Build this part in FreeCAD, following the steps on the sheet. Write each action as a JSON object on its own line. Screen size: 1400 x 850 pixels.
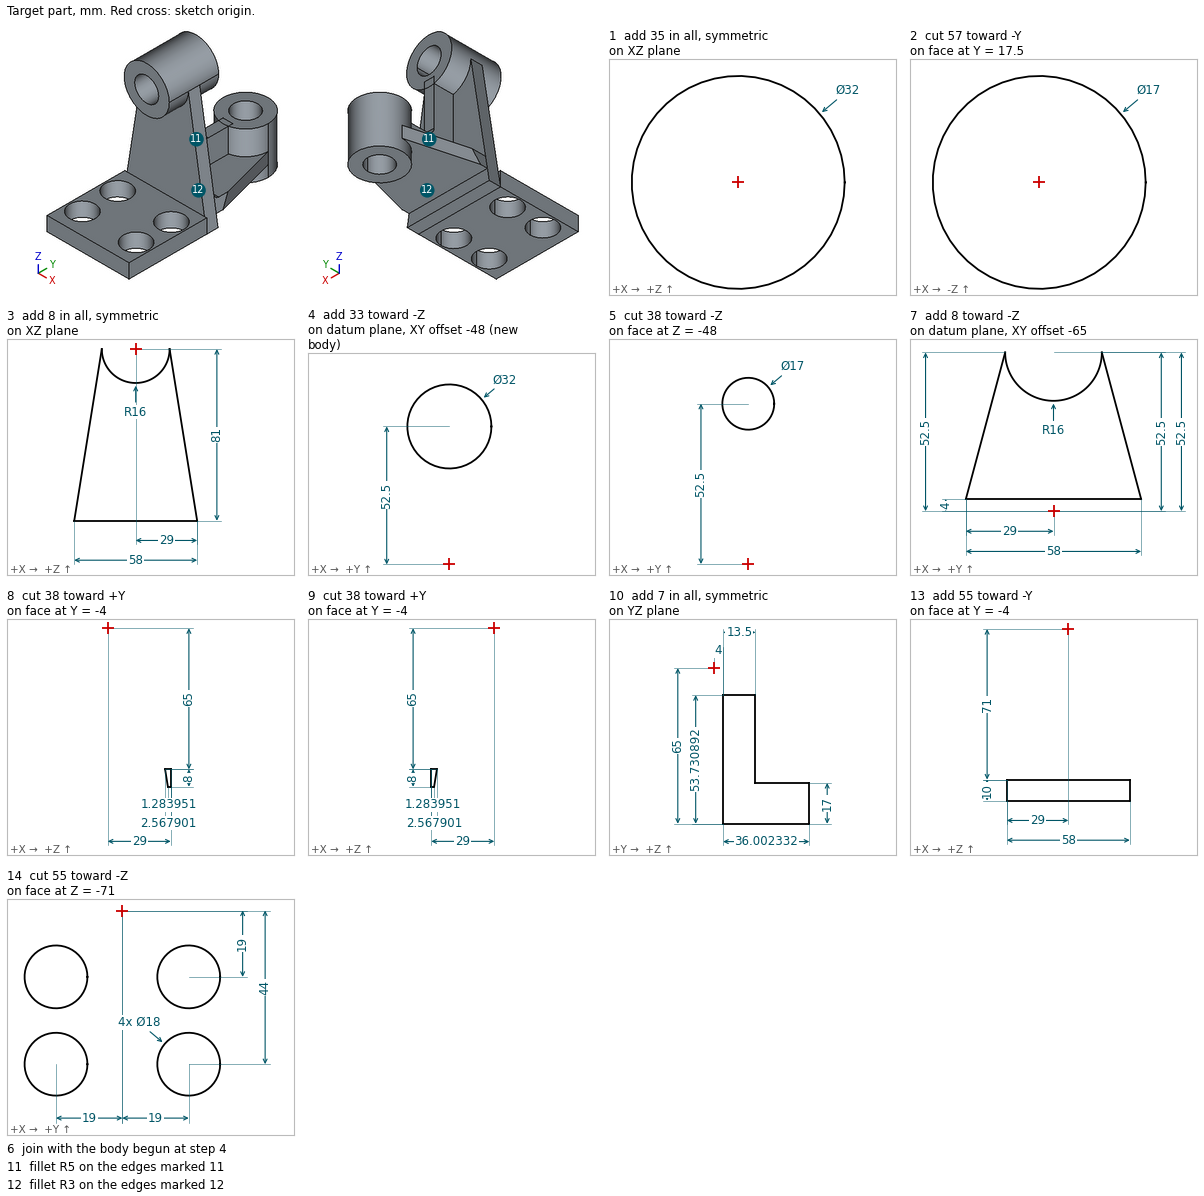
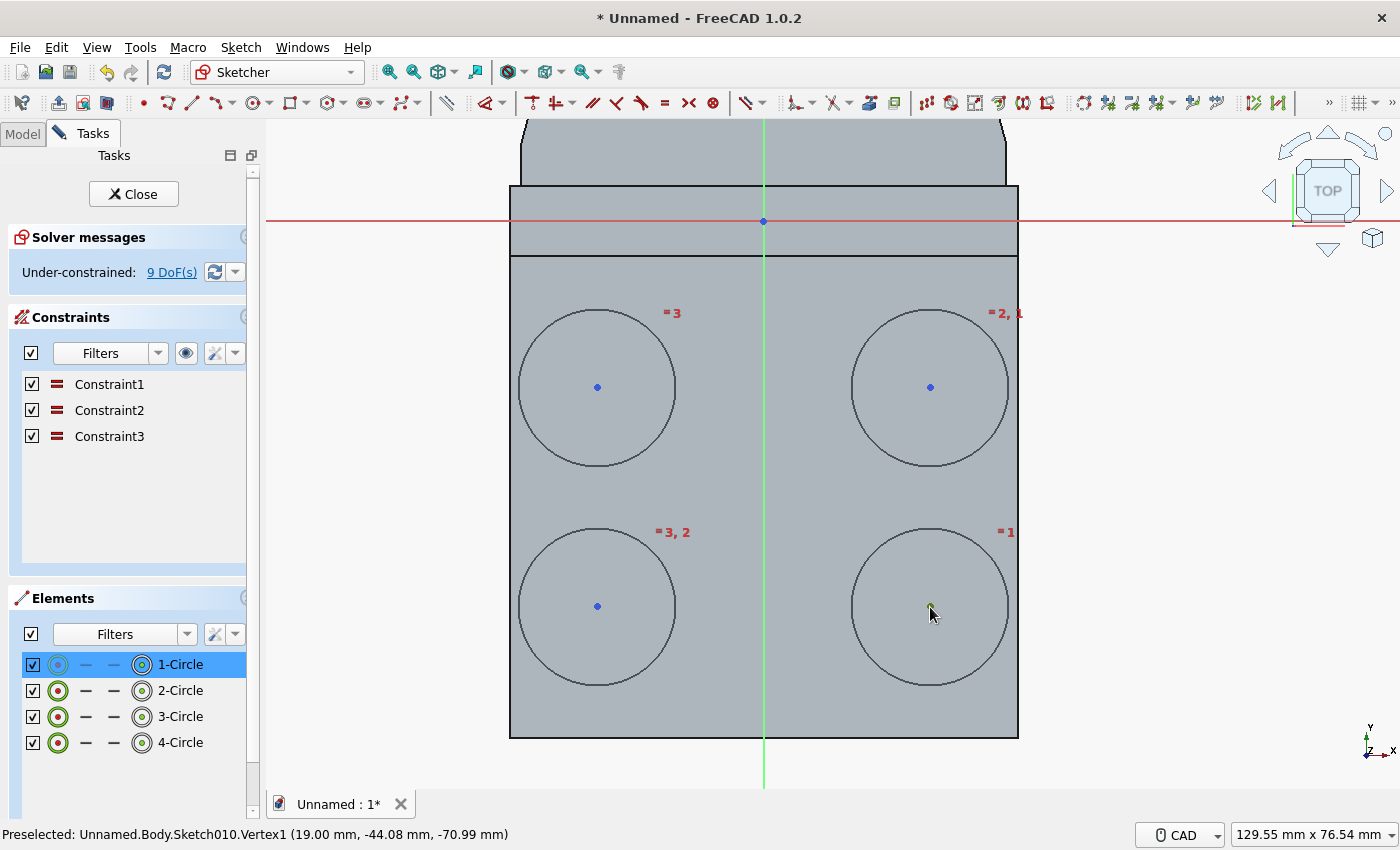
{"action": "left_click", "coordinate": [930, 388]}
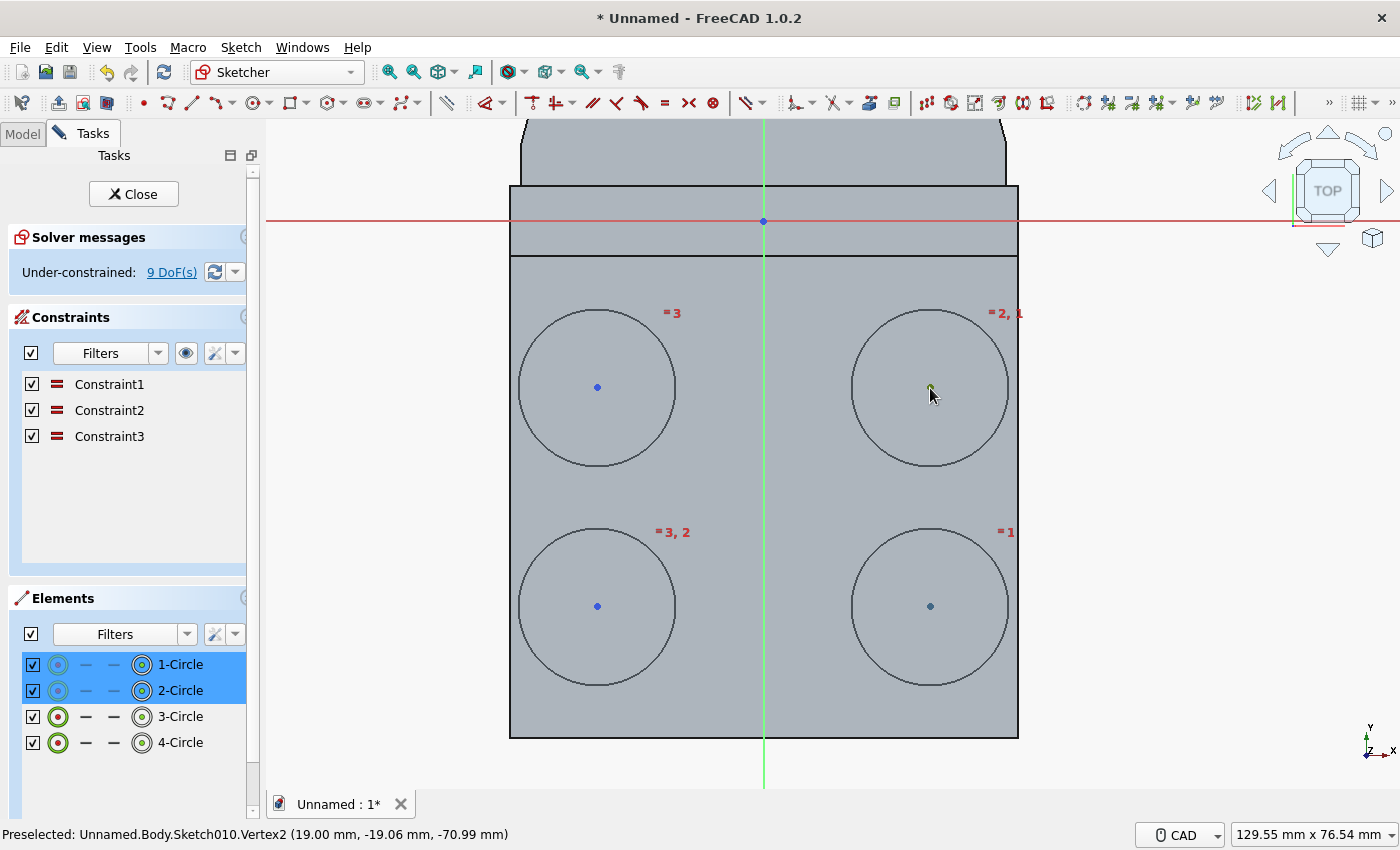
{"action": "left_click", "coordinate": [574, 104]}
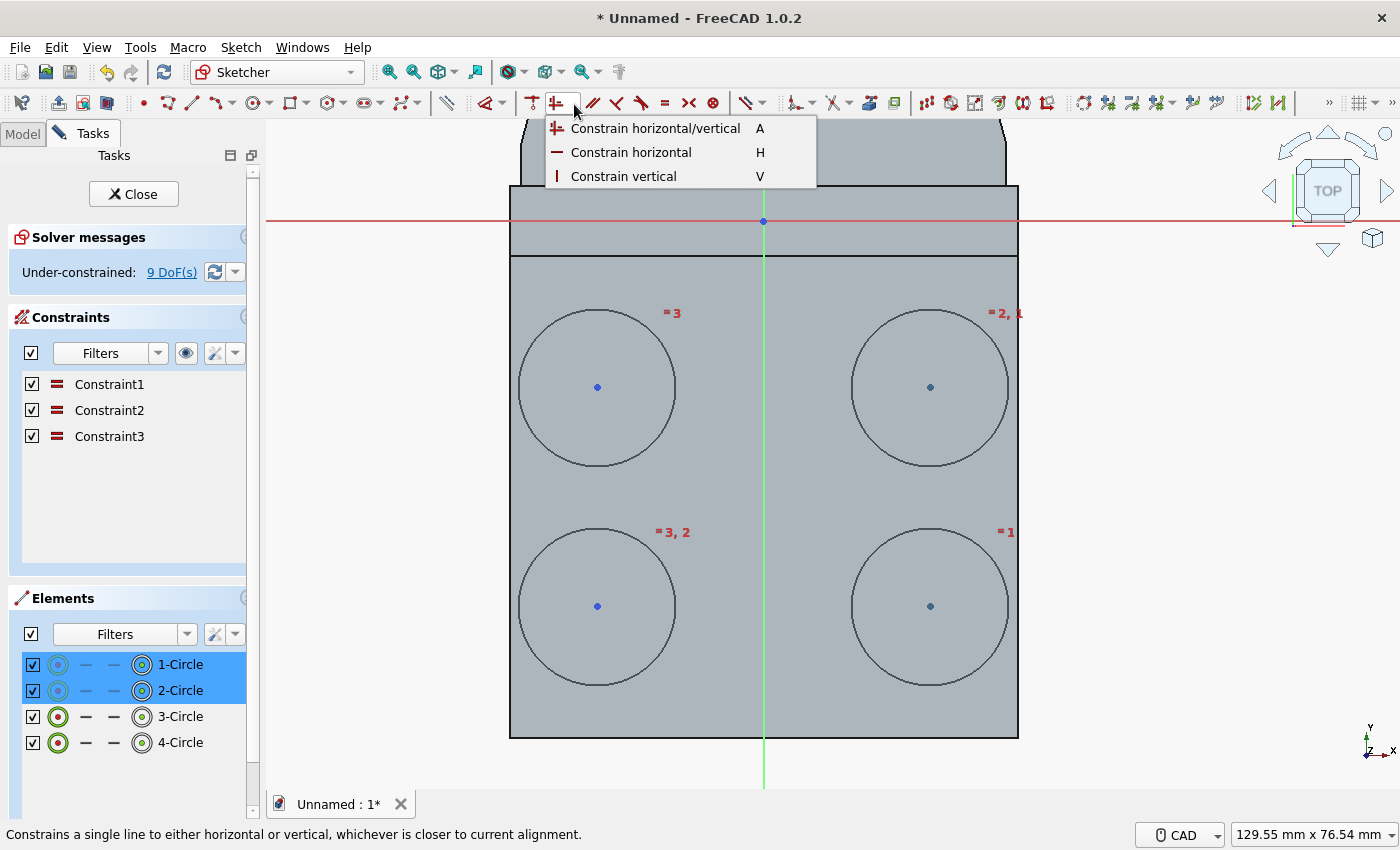
{"action": "left_click", "coordinate": [681, 176]}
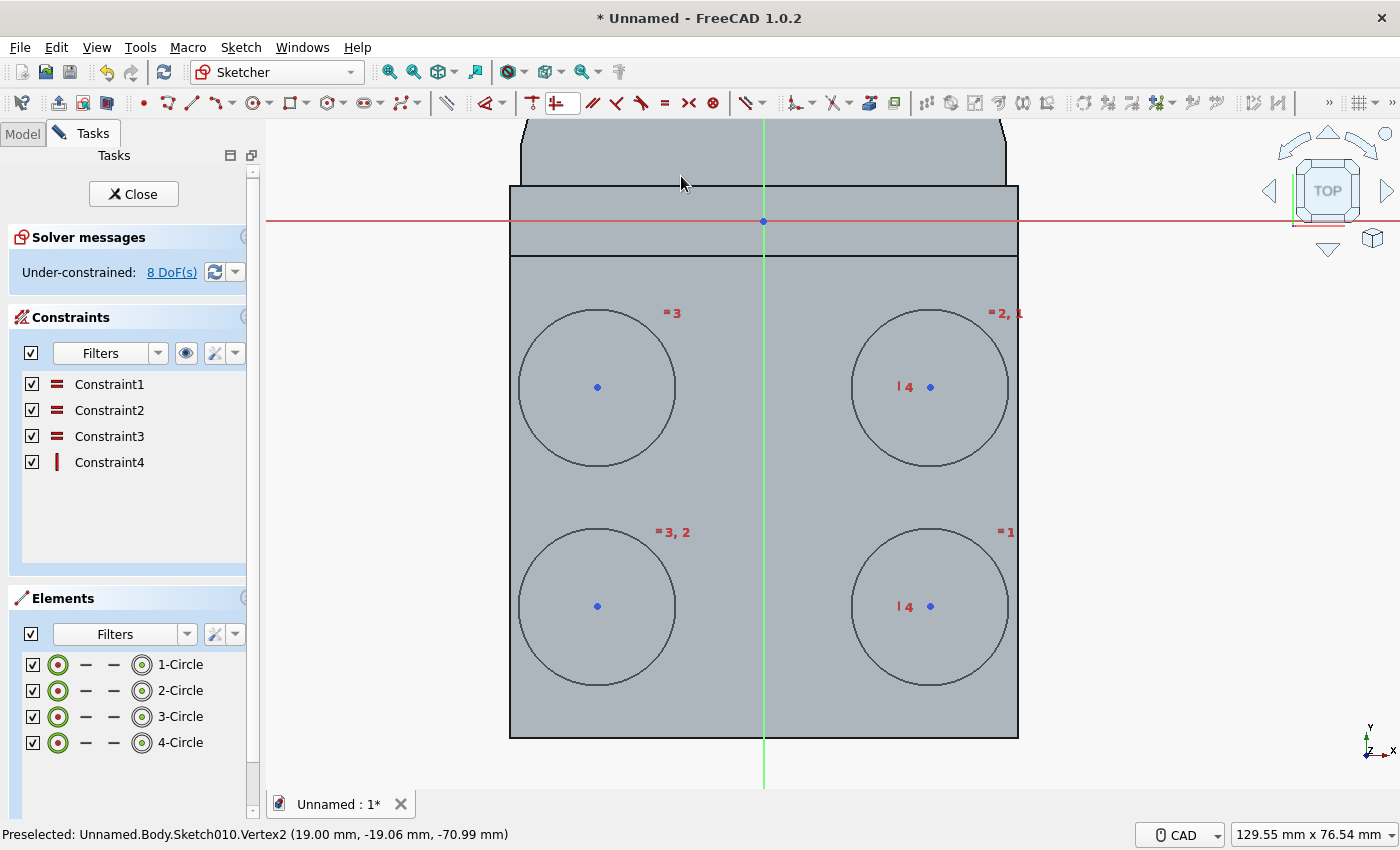
{"action": "left_click", "coordinate": [930, 607]}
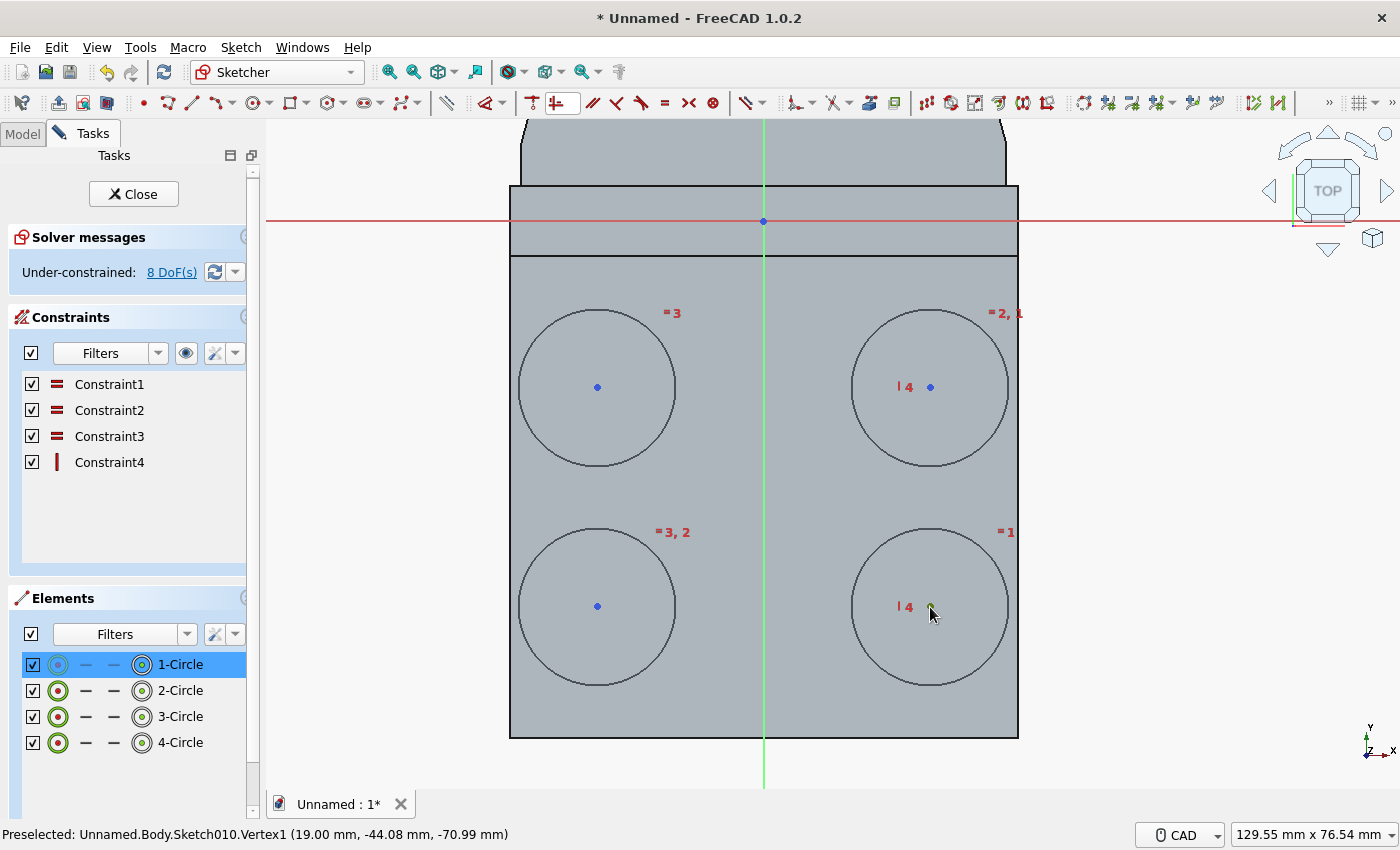
{"action": "left_click", "coordinate": [597, 607]}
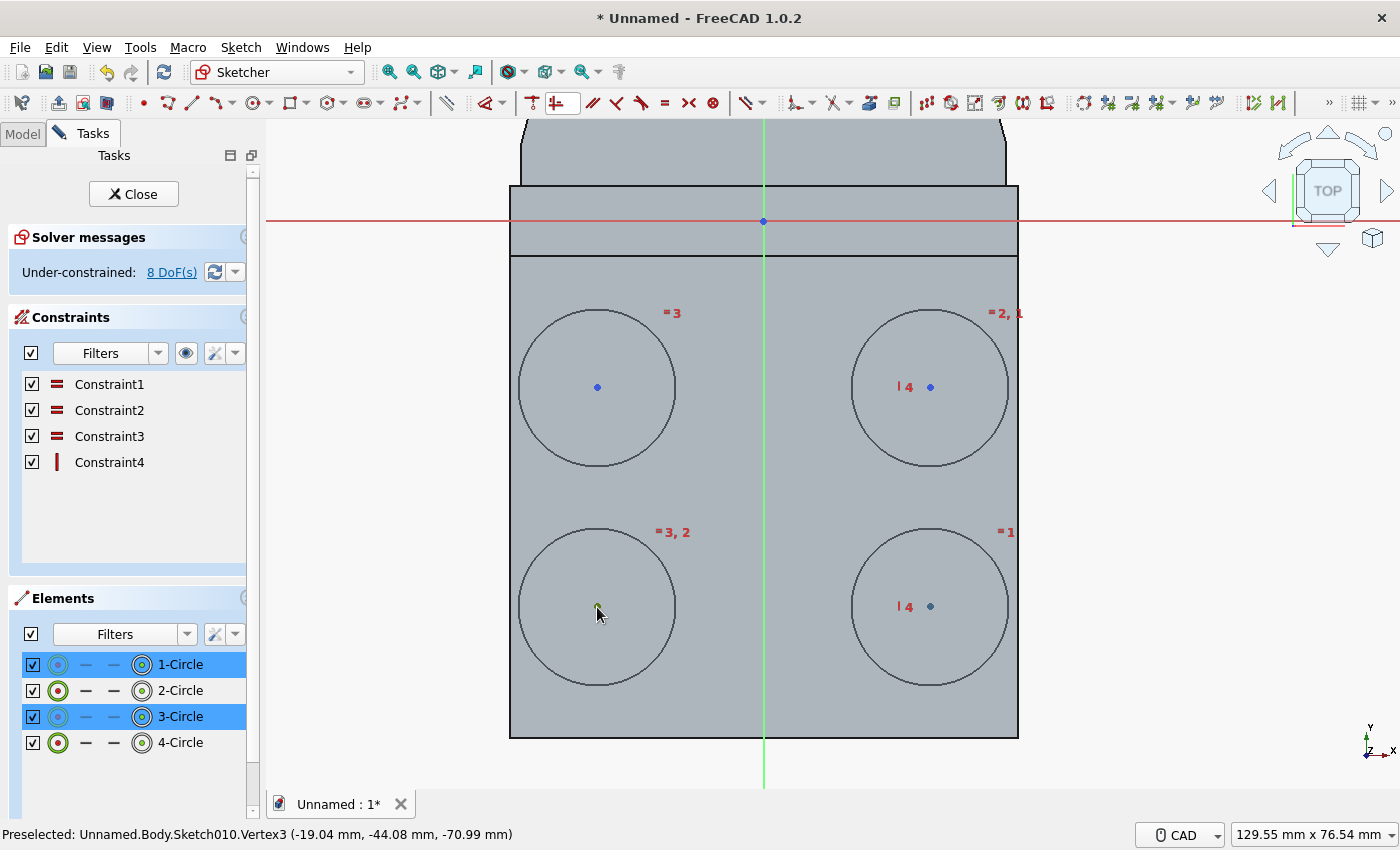
{"action": "key", "text": "h"}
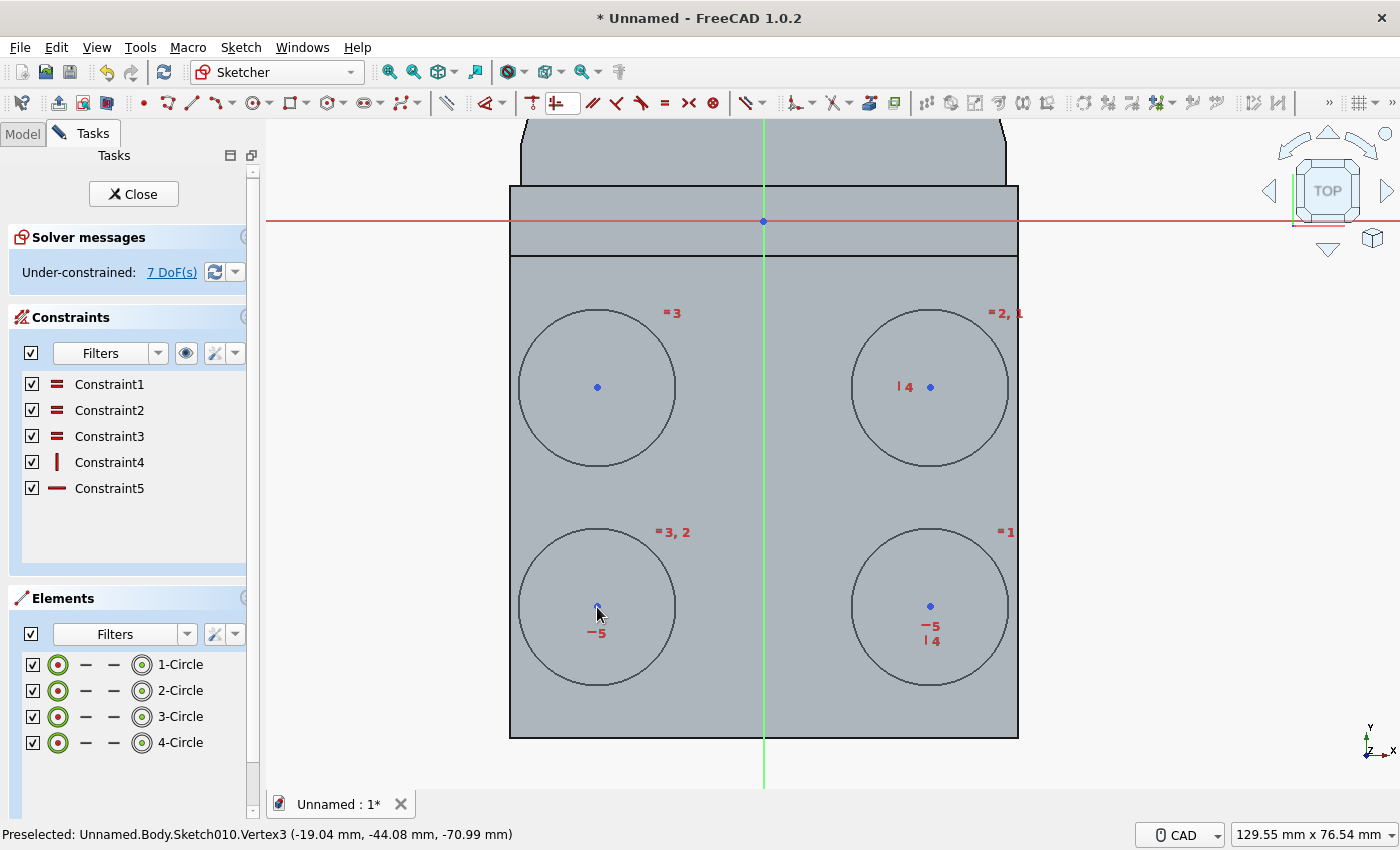
{"action": "left_click", "coordinate": [597, 607]}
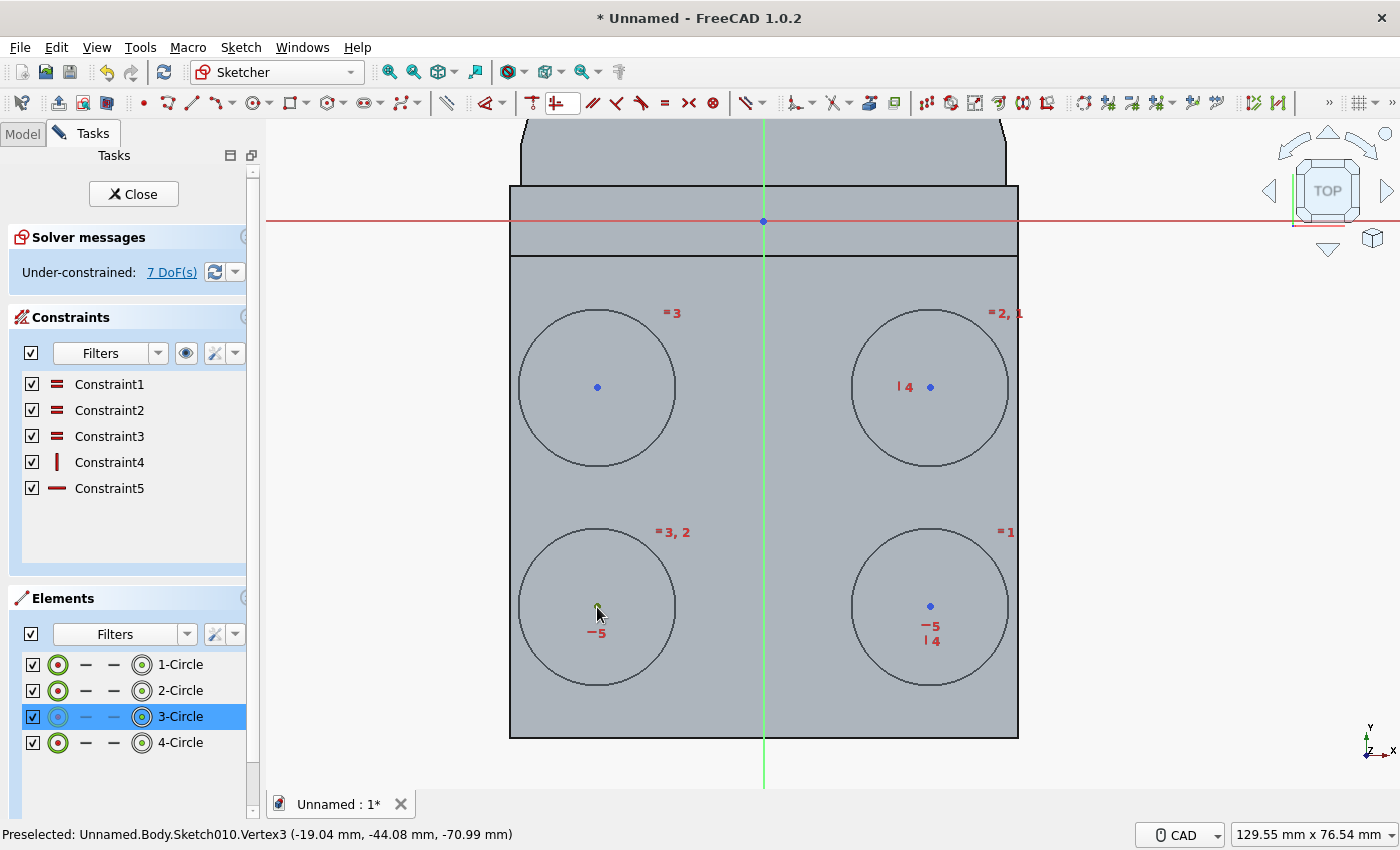
{"action": "left_click", "coordinate": [597, 388]}